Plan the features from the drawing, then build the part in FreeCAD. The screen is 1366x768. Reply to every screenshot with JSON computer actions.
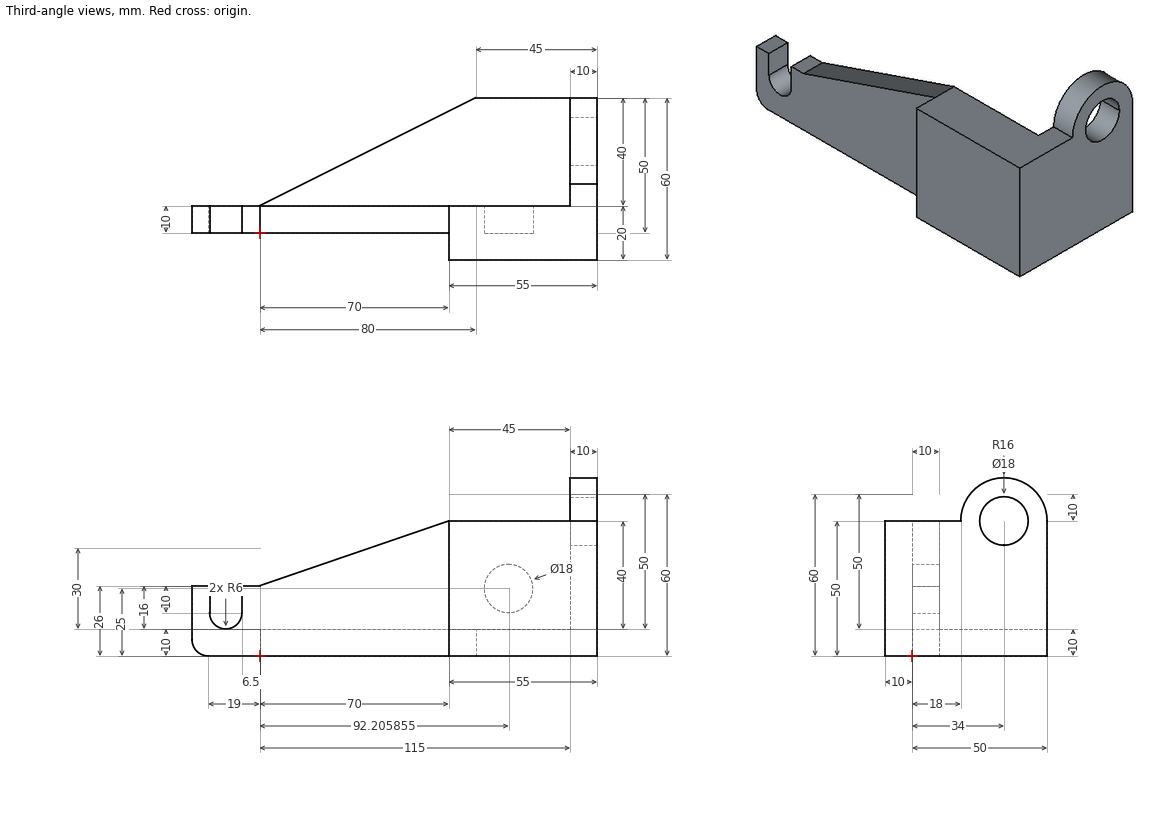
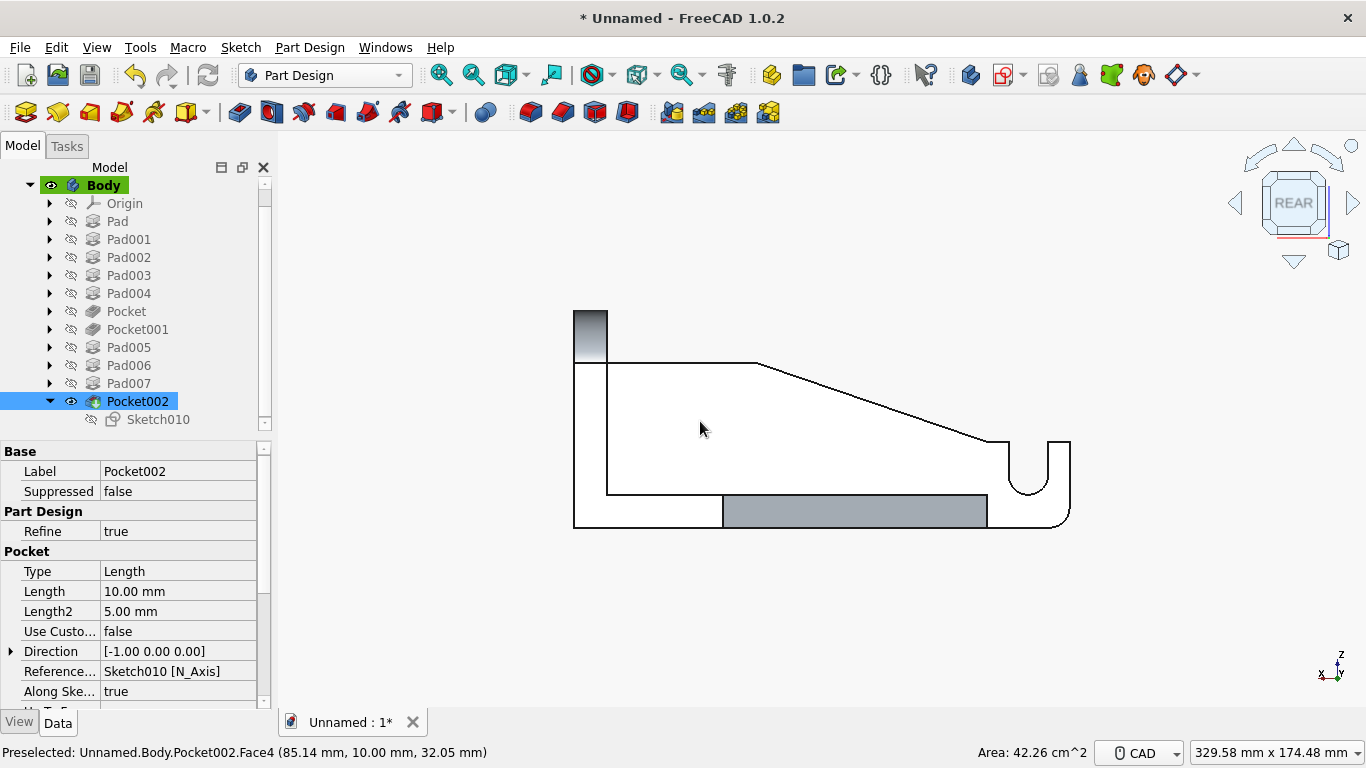
{"action": "left_click", "coordinate": [1004, 76]}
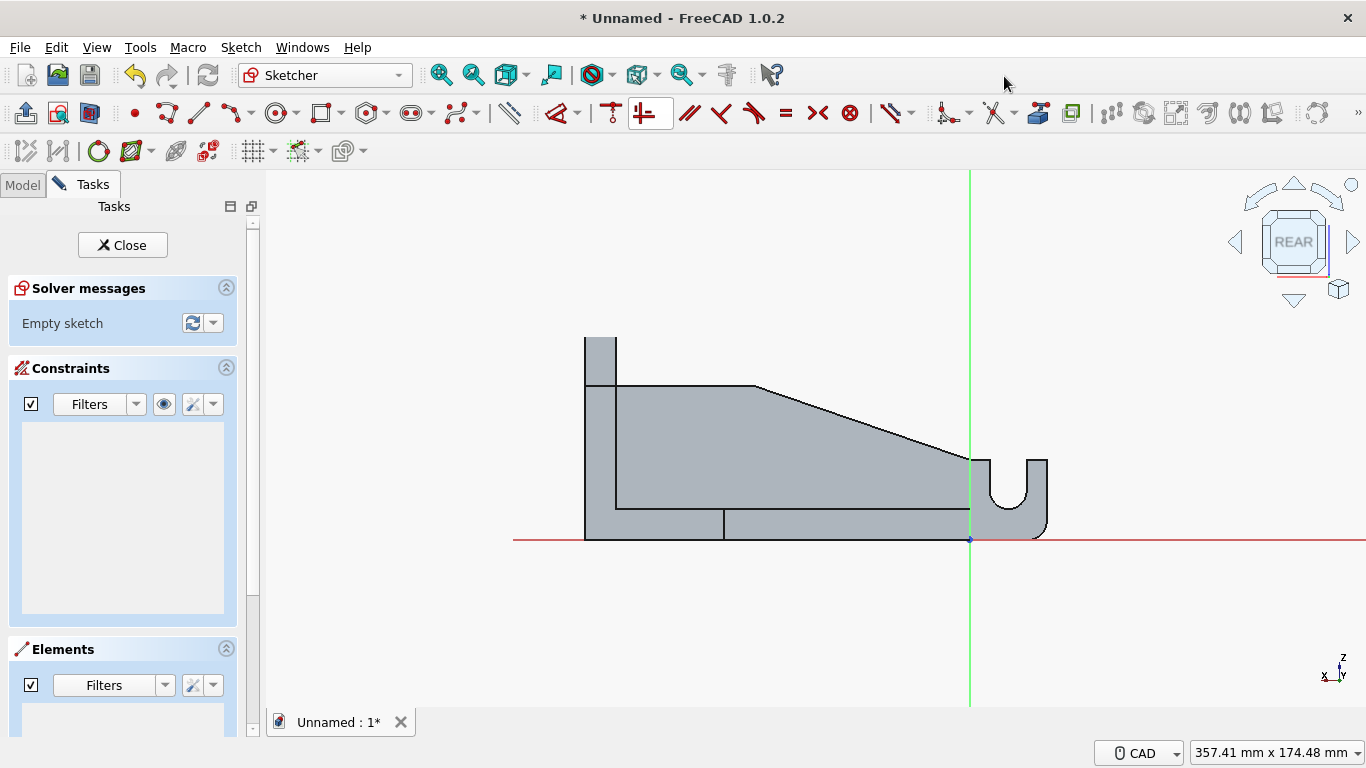
{"action": "scroll", "coordinate": [674, 468], "scroll_direction": "up", "scroll_amount": 9}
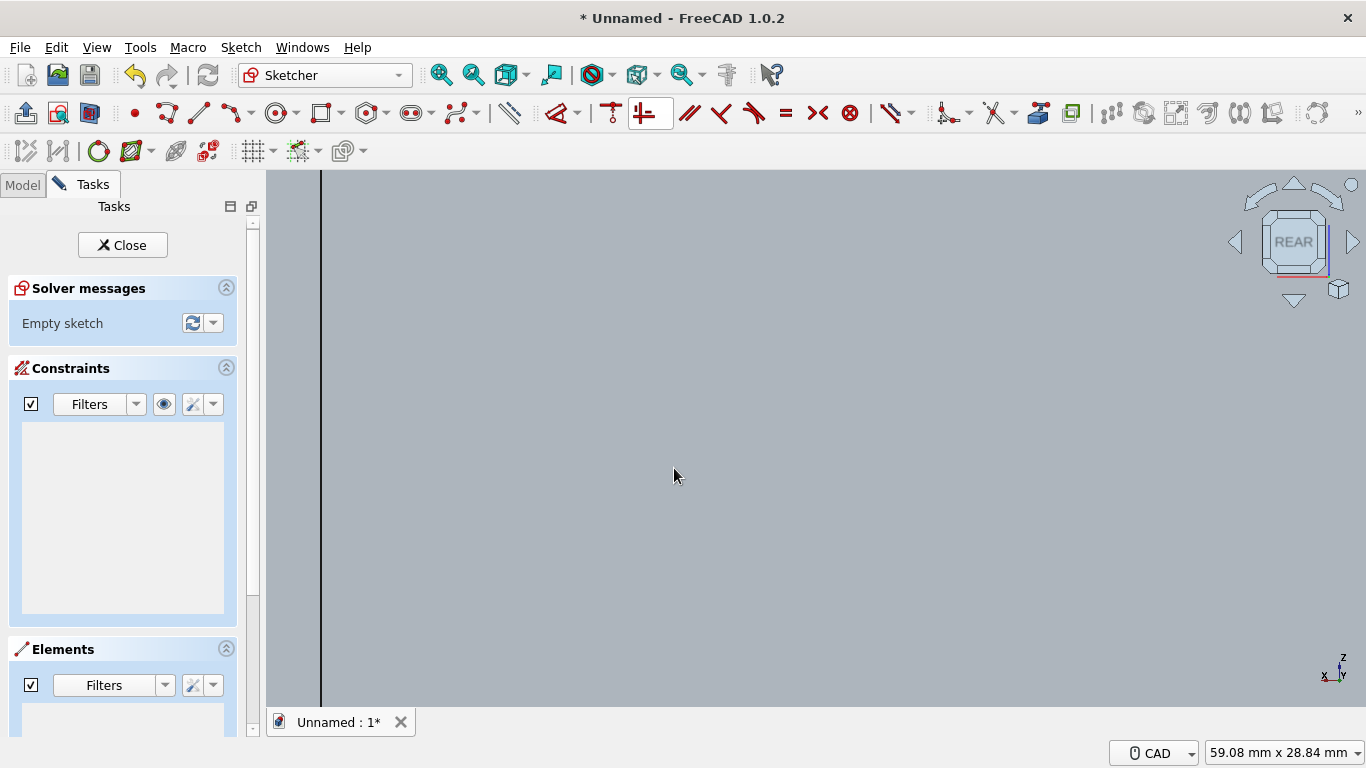
{"action": "left_click", "coordinate": [276, 114]}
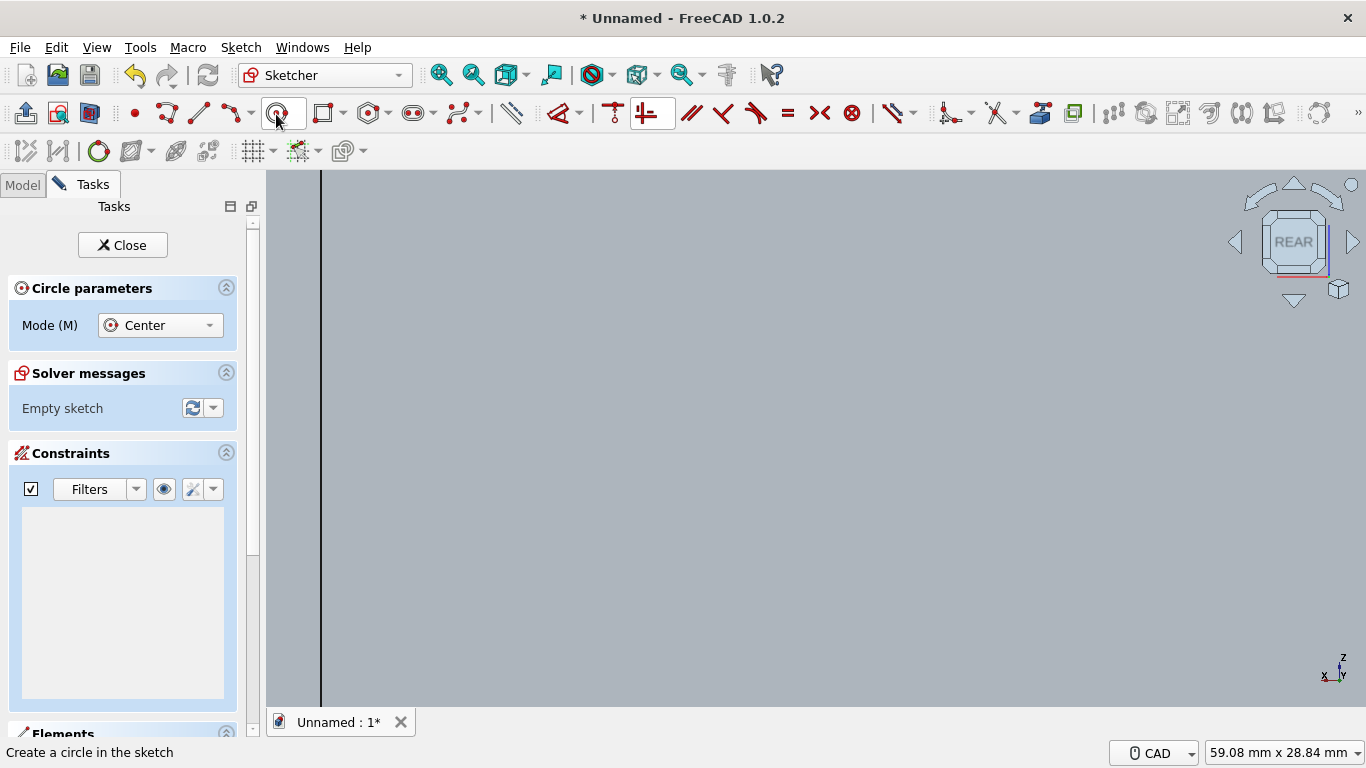
{"action": "left_click", "coordinate": [745, 435]}
{"action": "left_click", "coordinate": [864, 316]}
{"action": "key", "text": "Escape"}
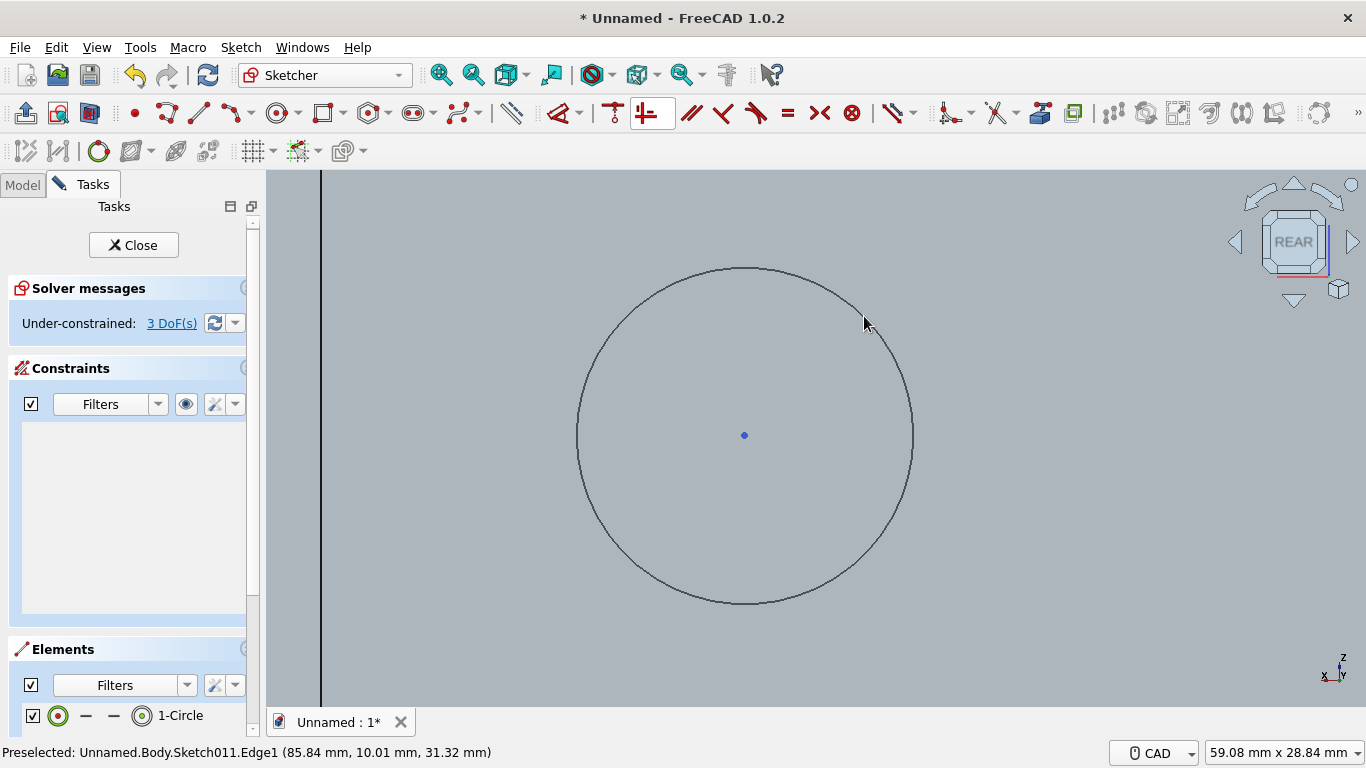
{"action": "left_click", "coordinate": [558, 114]}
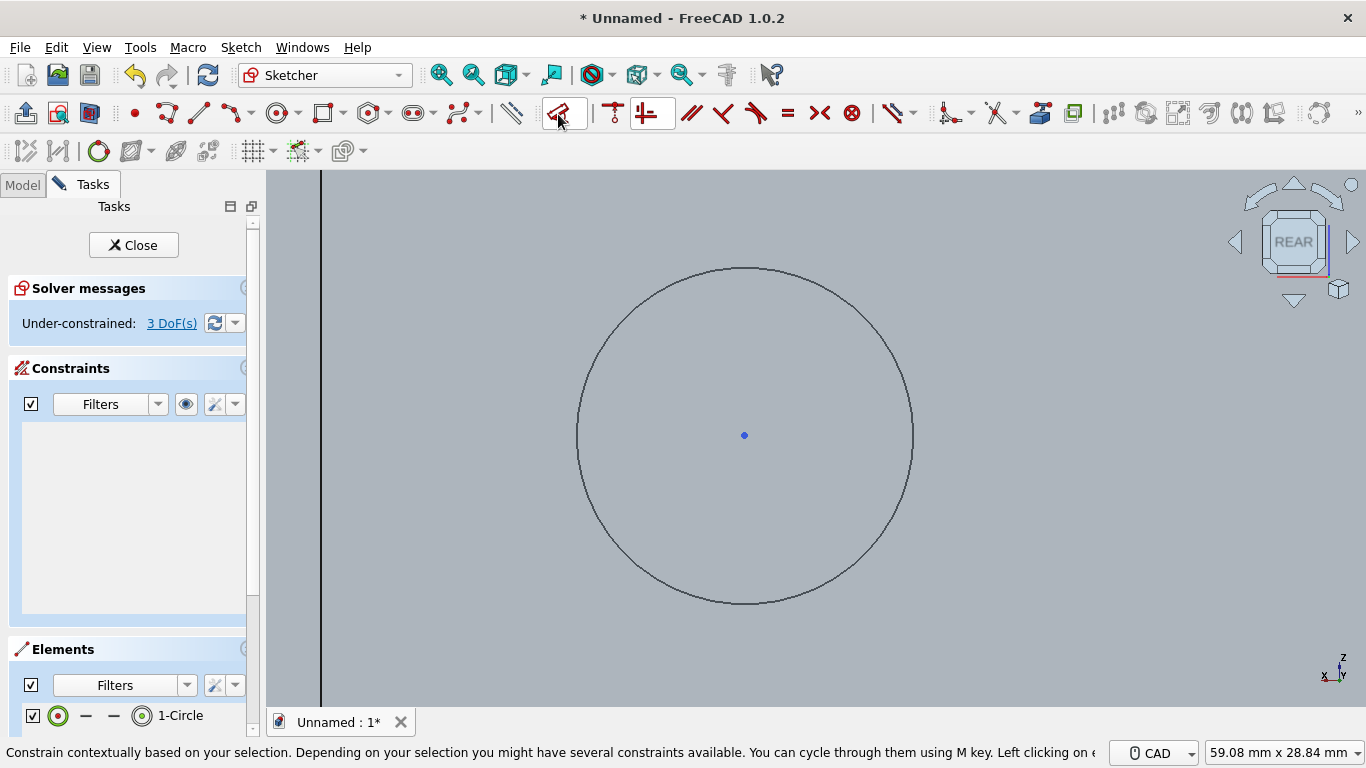
{"action": "left_click", "coordinate": [864, 317]}
{"action": "left_click", "coordinate": [887, 294]}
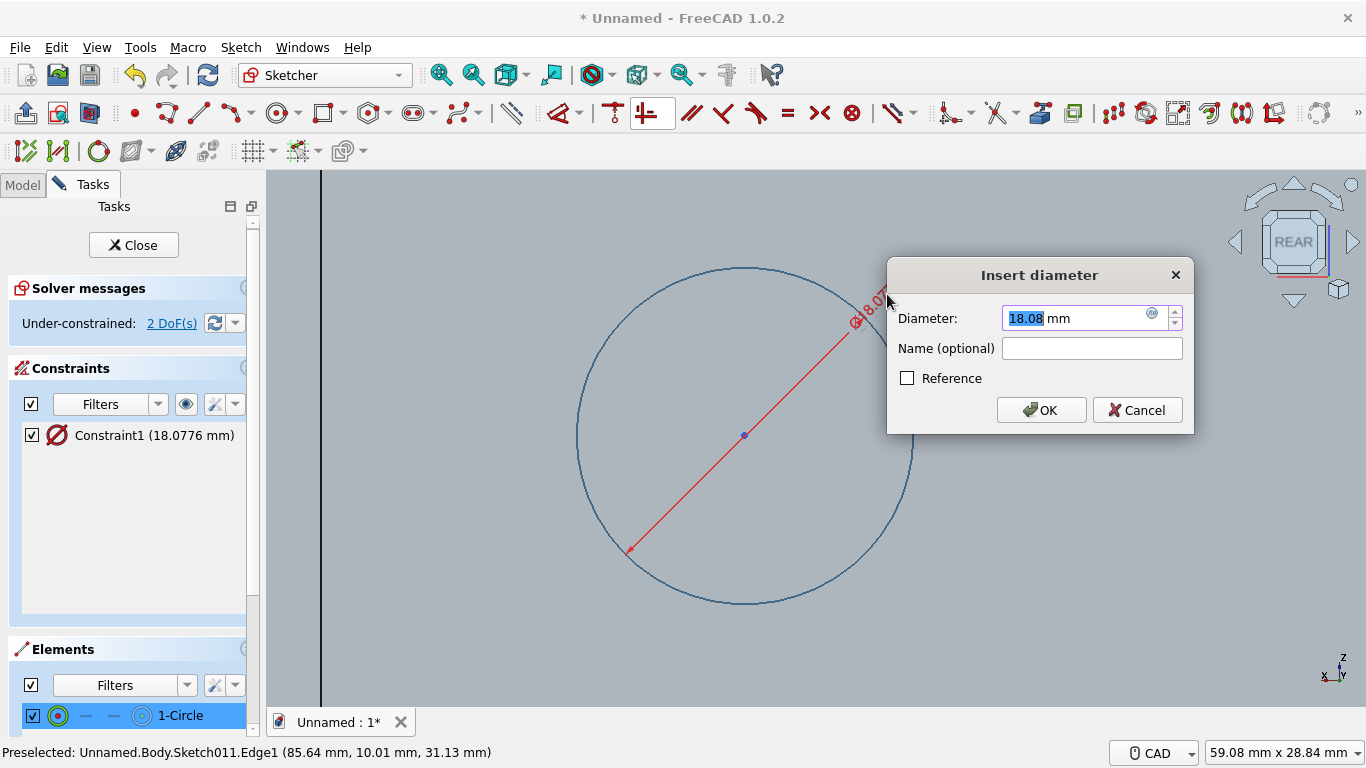
{"action": "type", "text": "18"}
{"action": "key", "text": "Return"}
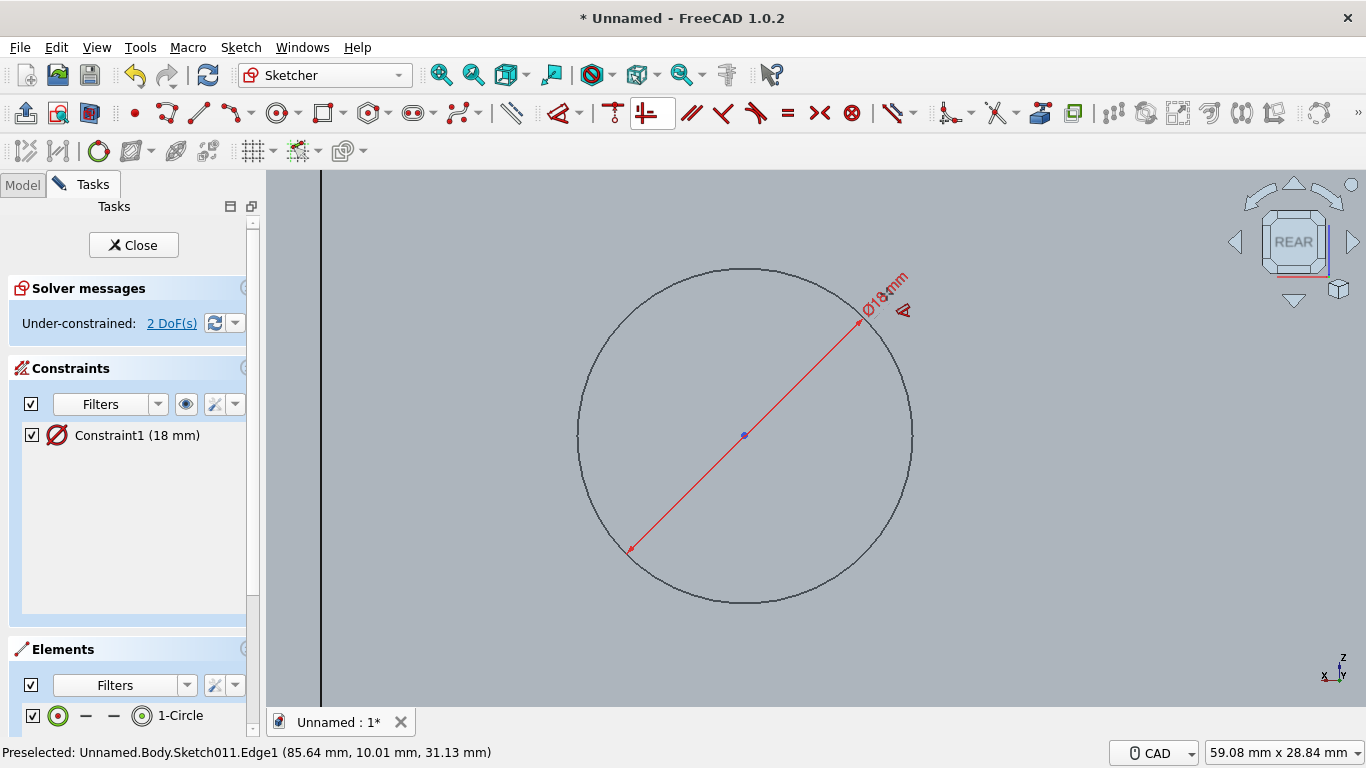
{"action": "left_click", "coordinate": [745, 436]}
{"action": "left_click", "coordinate": [711, 558]}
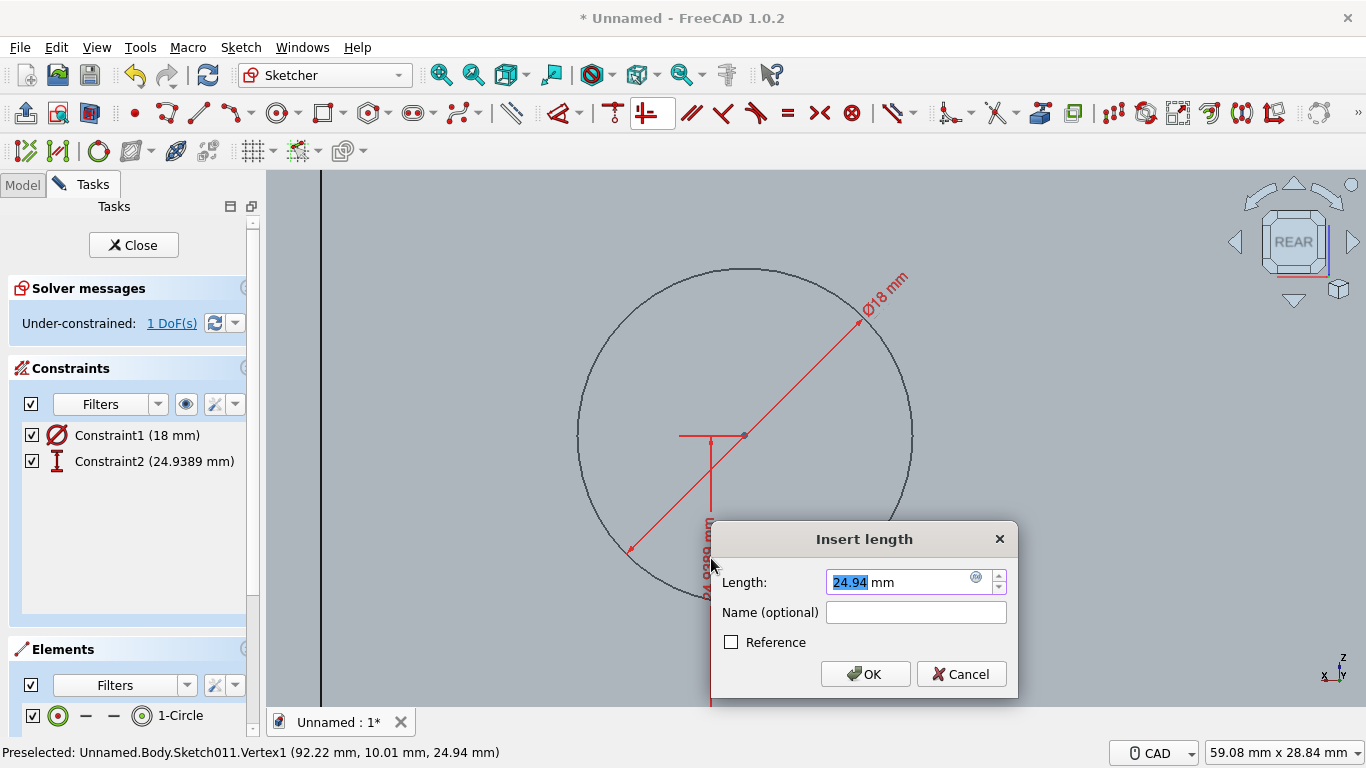
{"action": "type", "text": "25"}
{"action": "key", "text": "Return"}